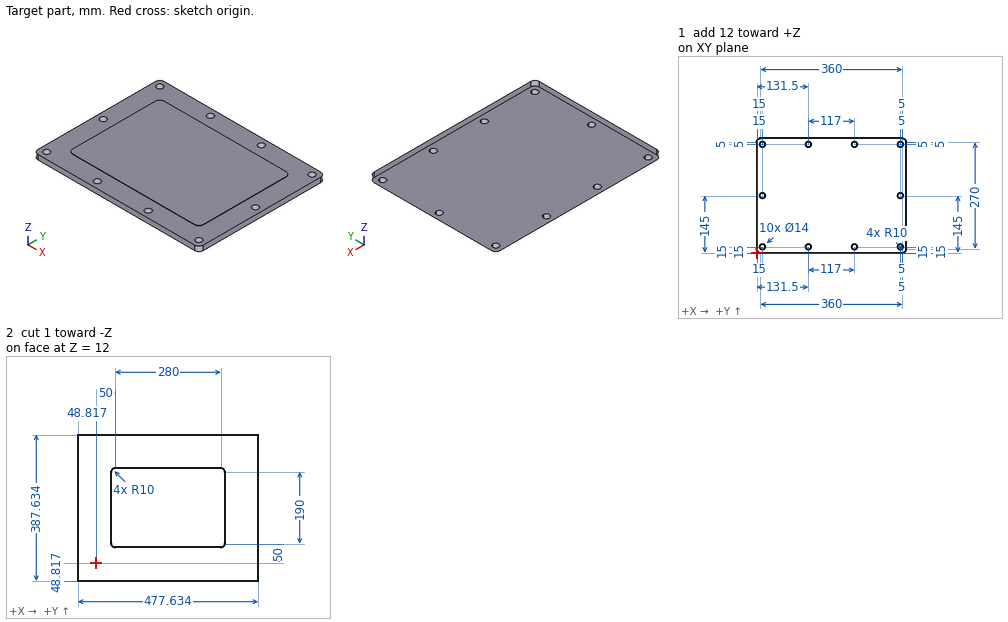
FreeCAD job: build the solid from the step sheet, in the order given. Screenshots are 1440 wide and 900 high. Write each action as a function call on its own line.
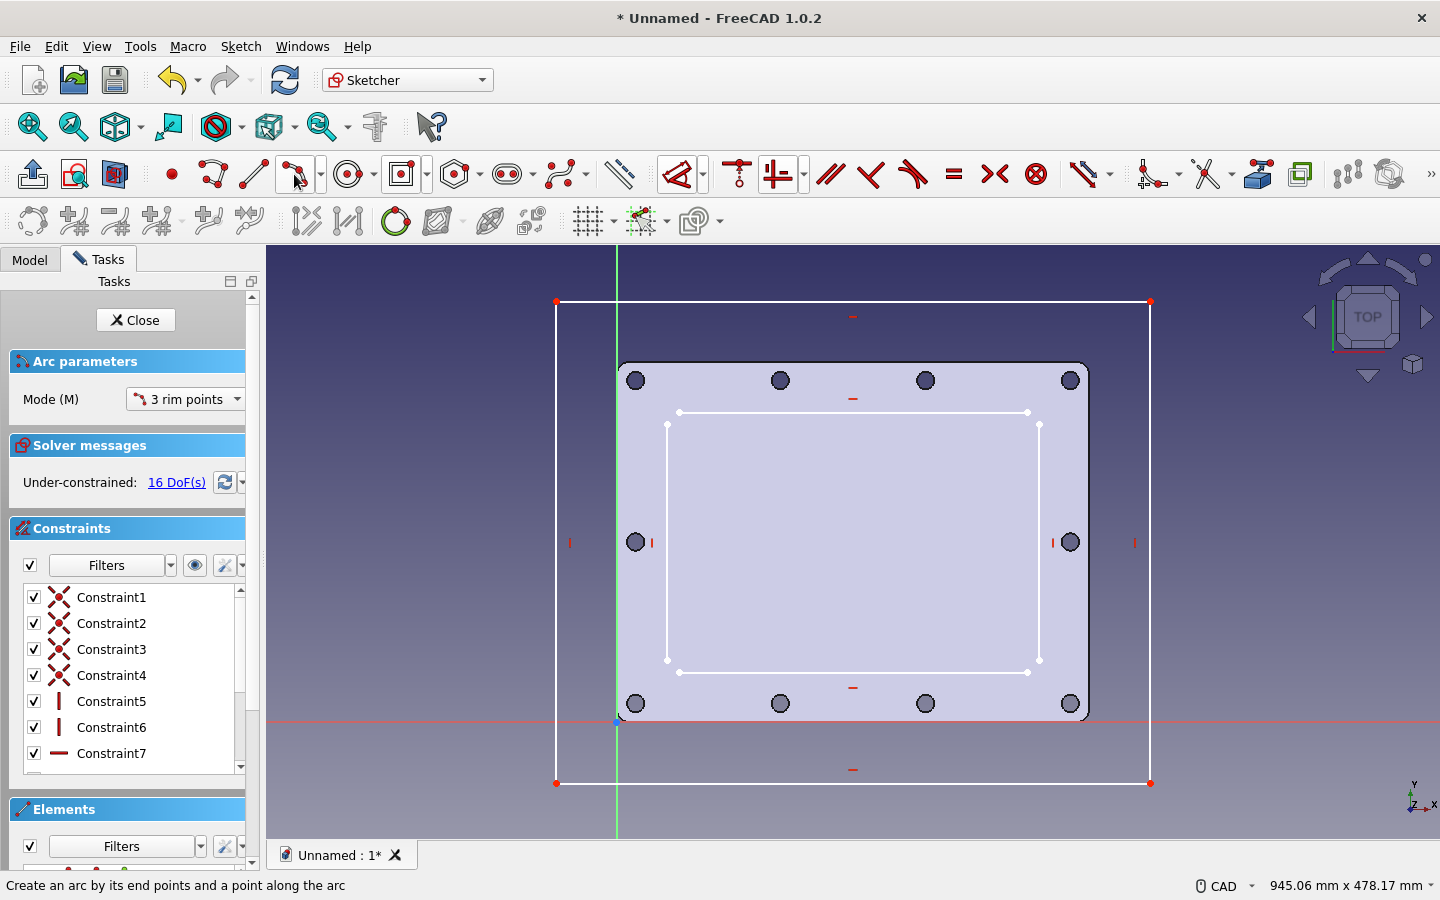
click(1027, 413)
click(1039, 425)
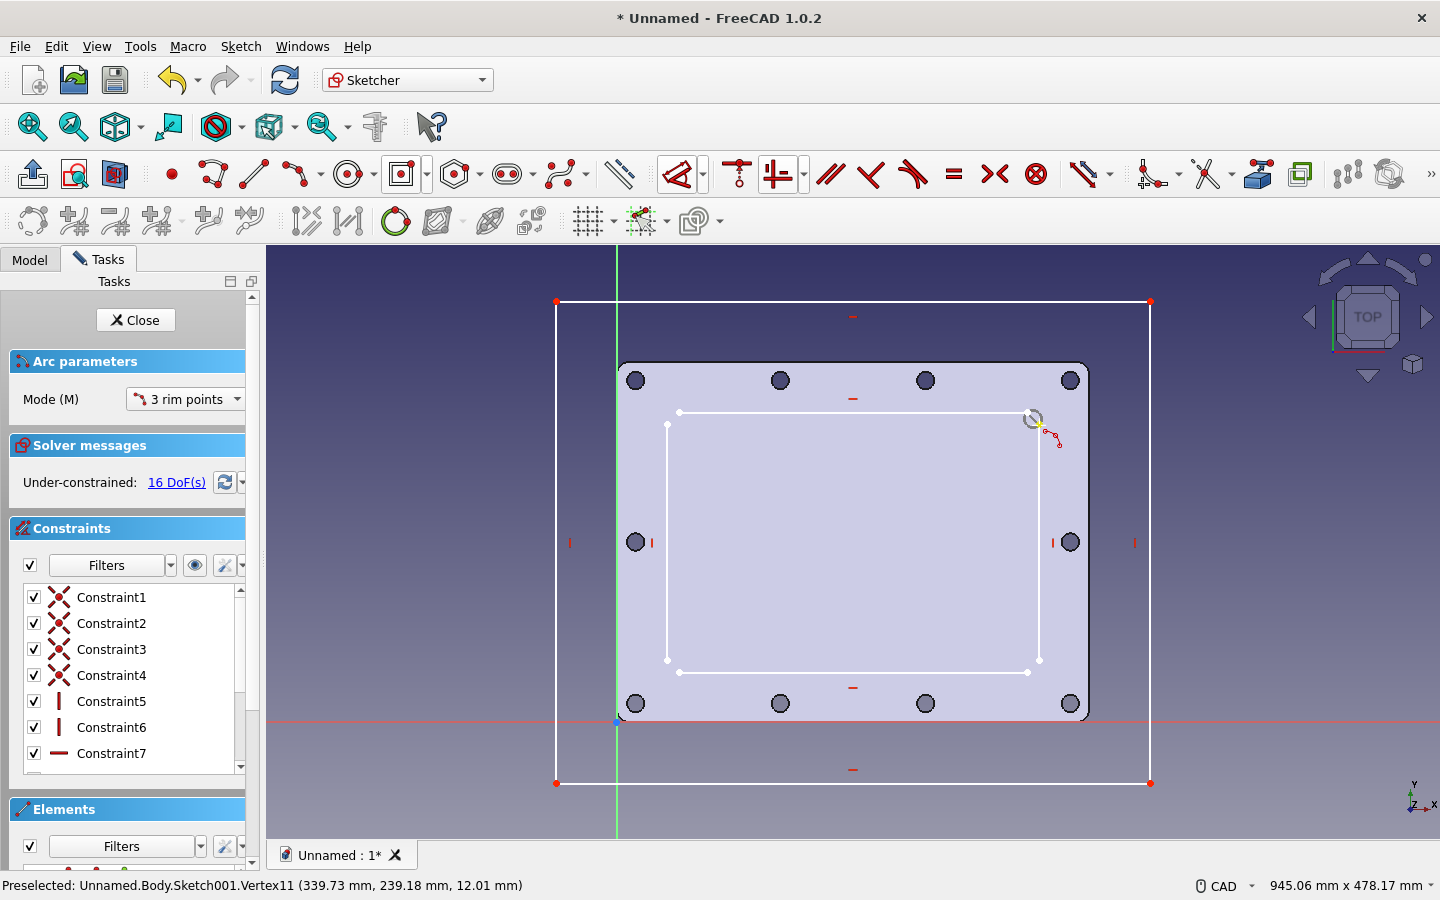
scroll(1036, 415, up, 8)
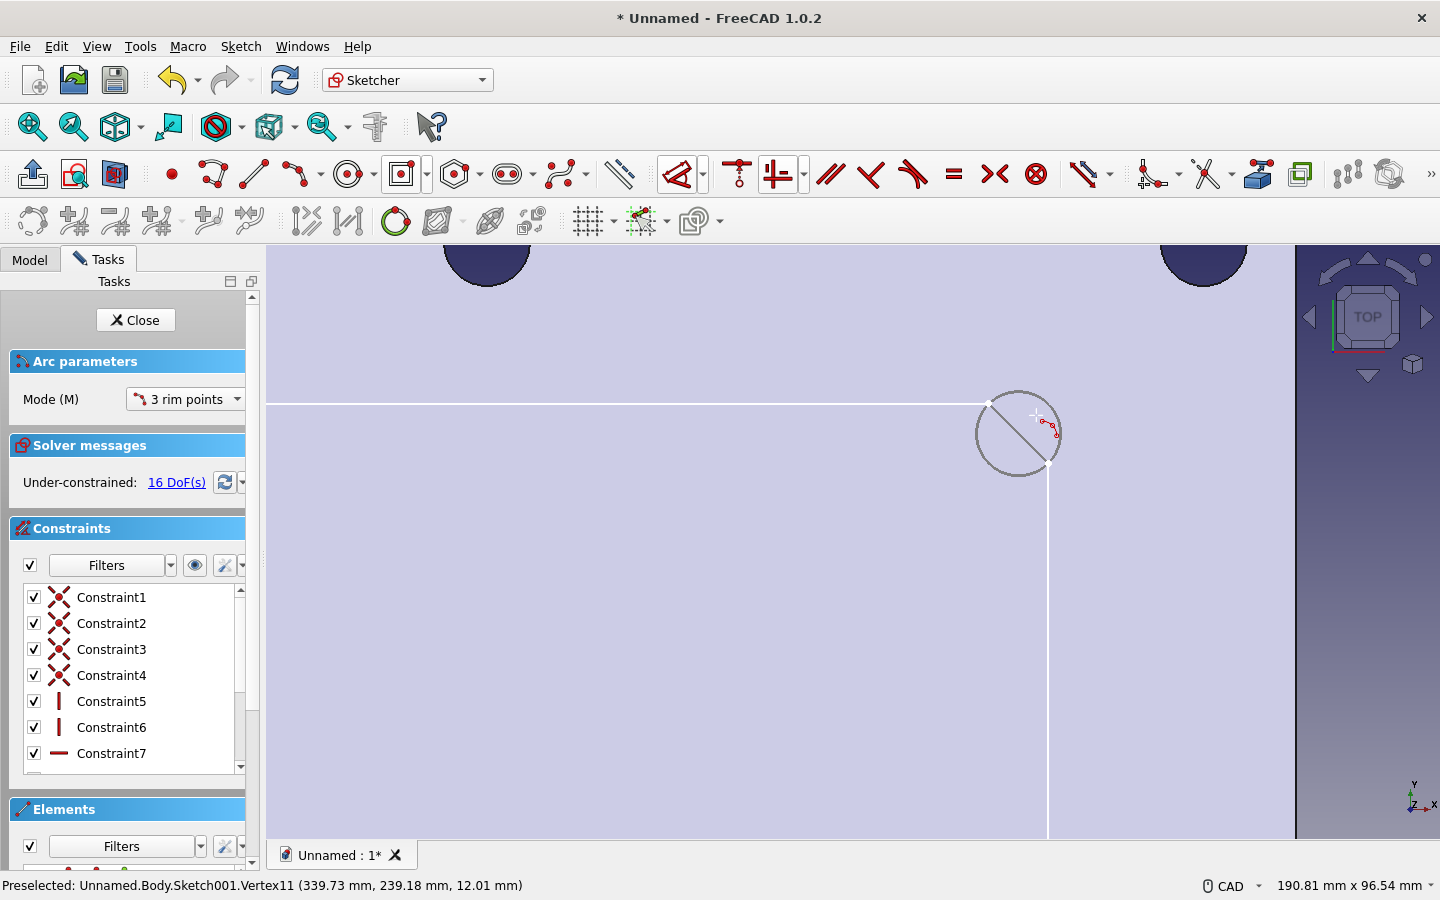
click(1032, 415)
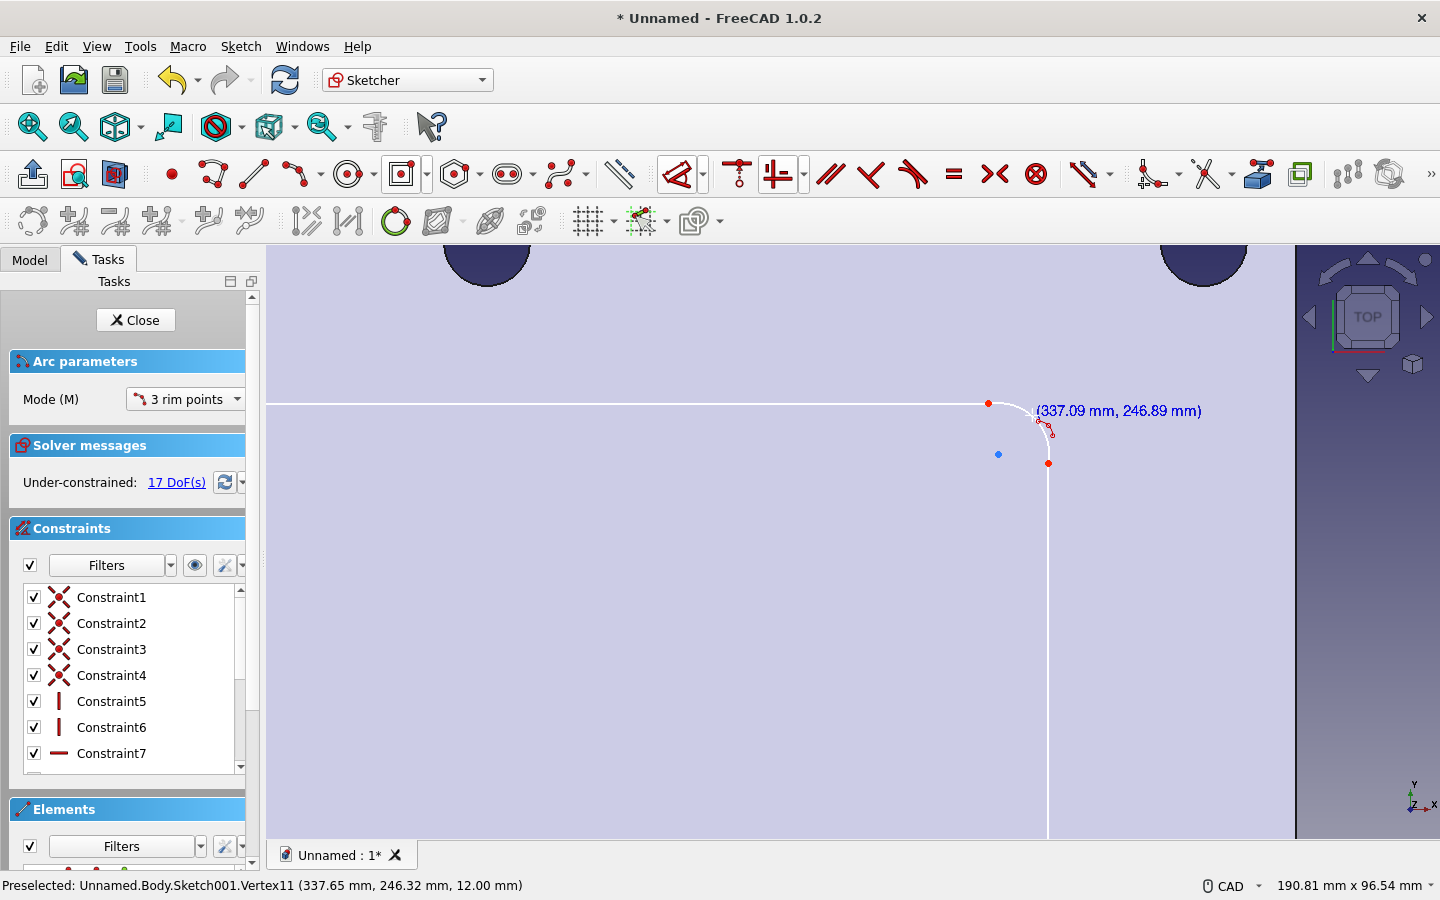
scroll(915, 443, down, 9)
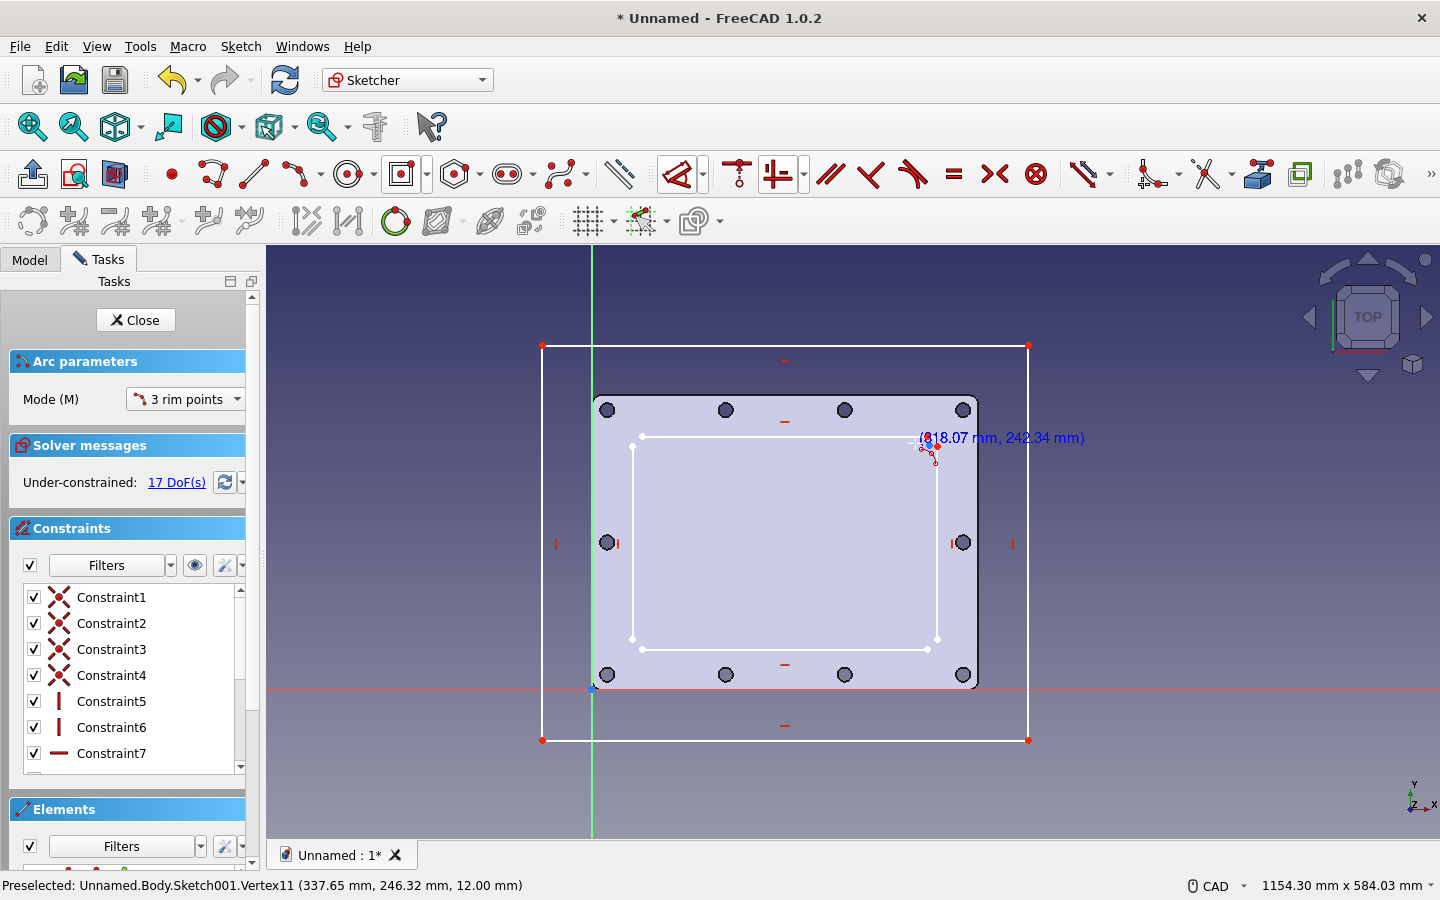
click(937, 640)
click(928, 650)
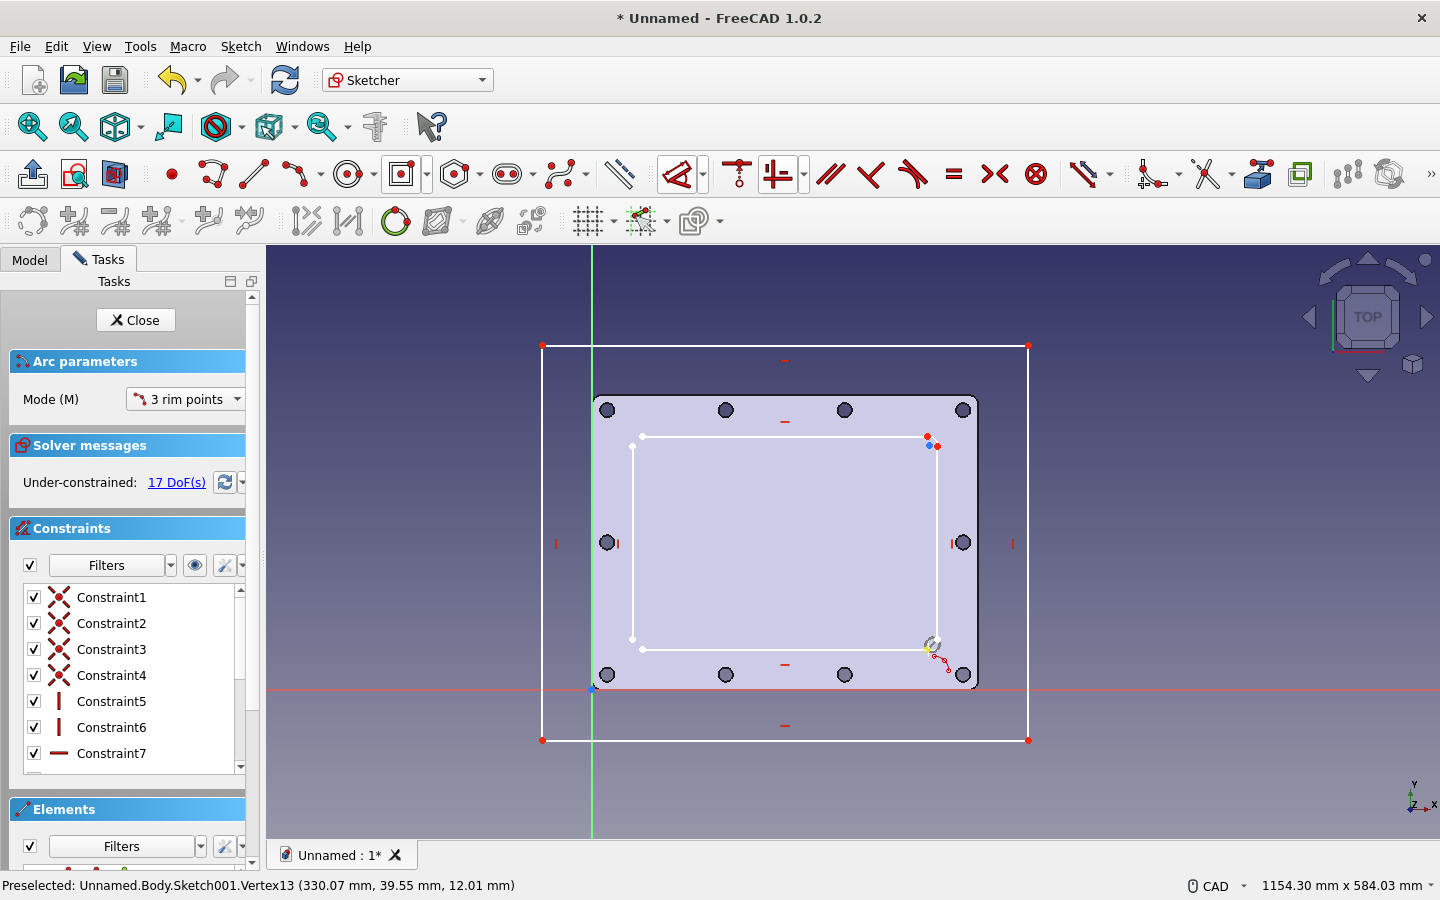
scroll(935, 646, up, 9)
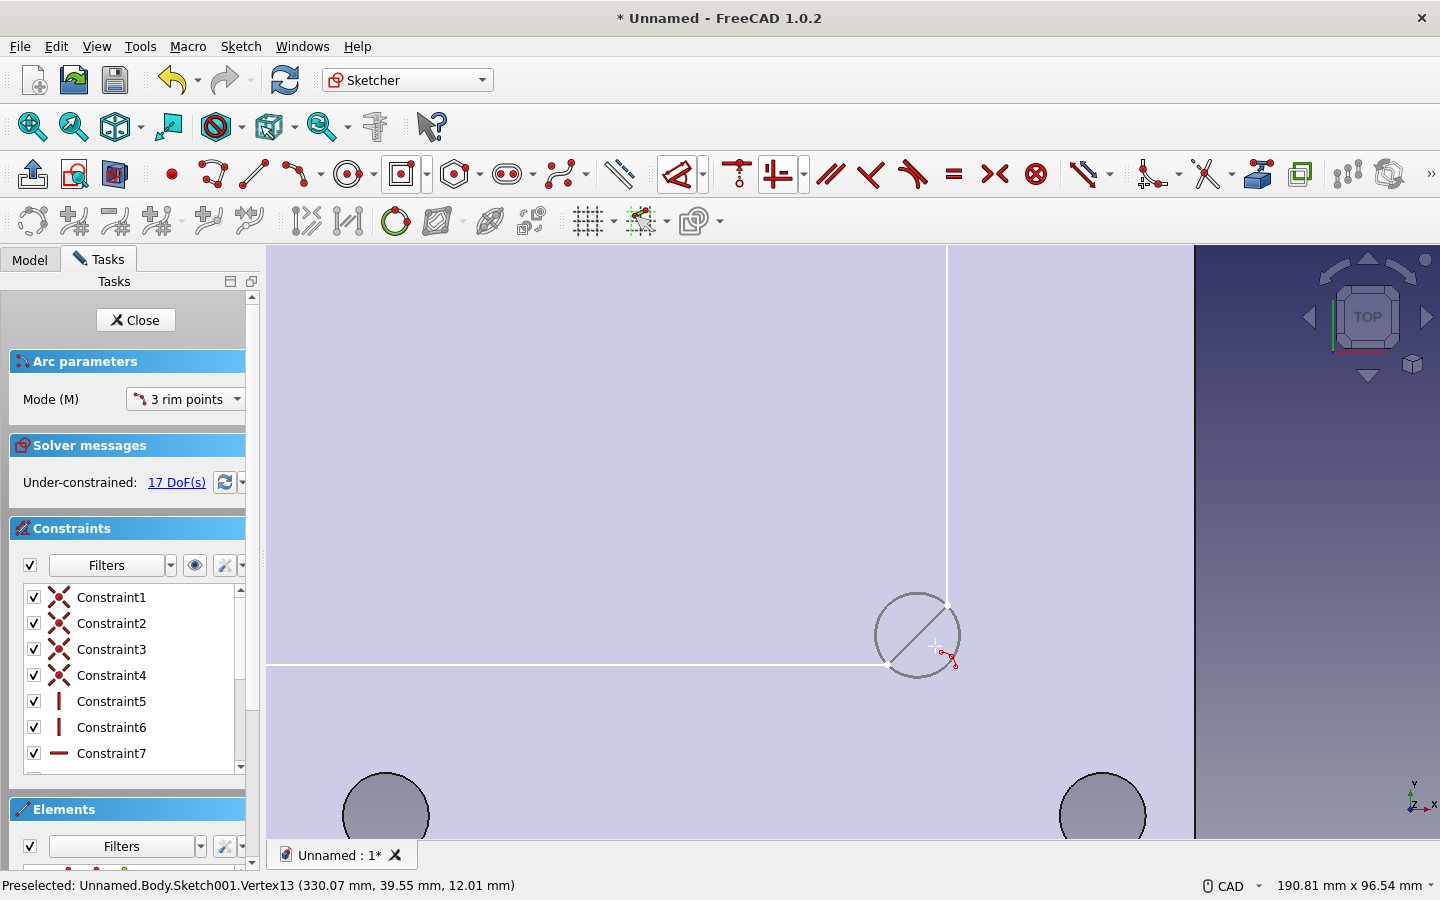
click(931, 644)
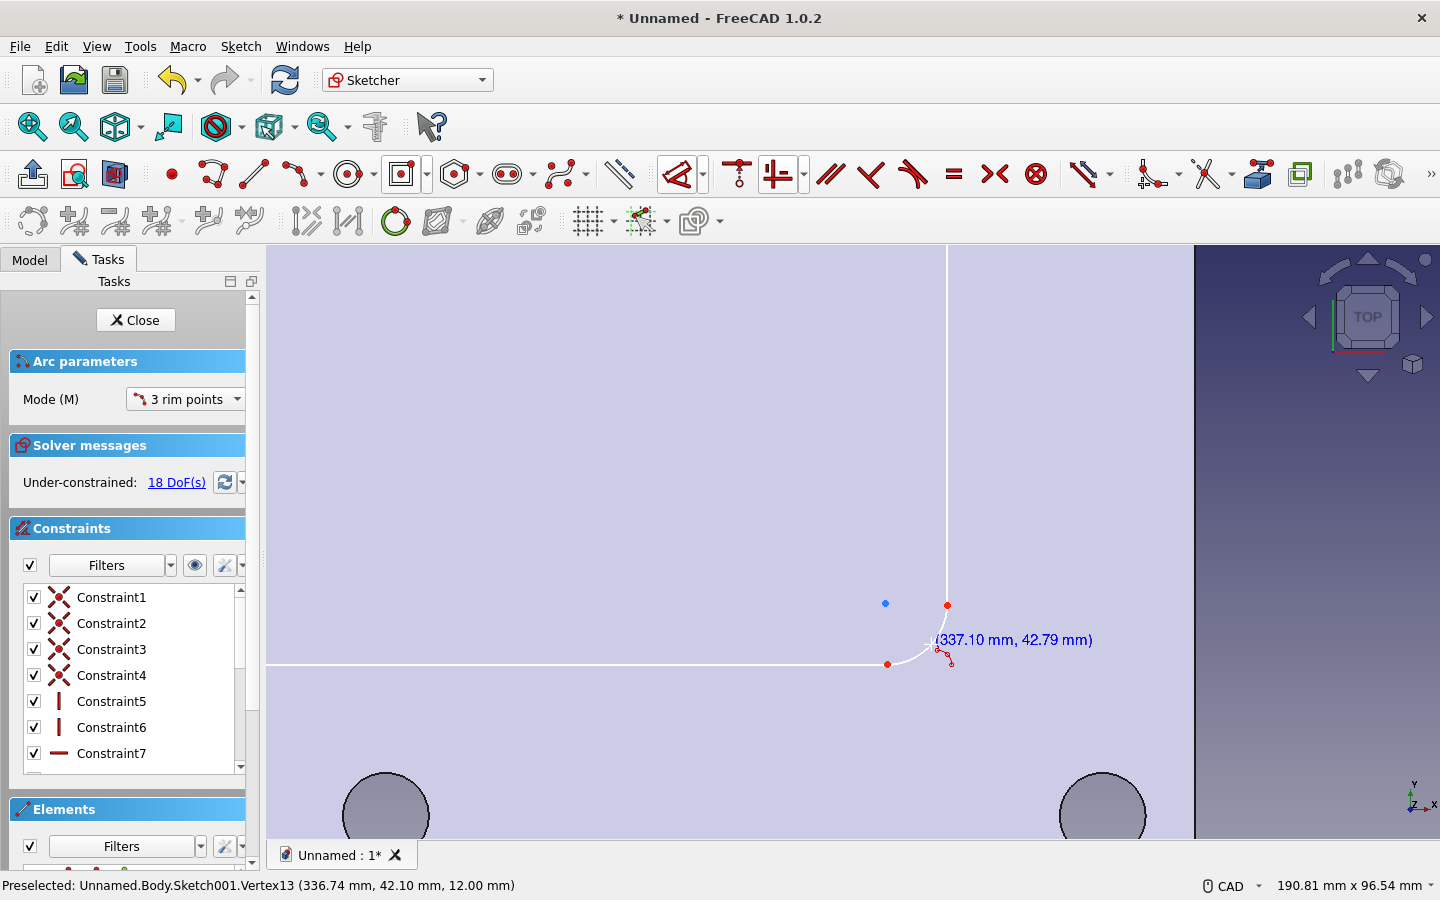
scroll(935, 646, down, 9)